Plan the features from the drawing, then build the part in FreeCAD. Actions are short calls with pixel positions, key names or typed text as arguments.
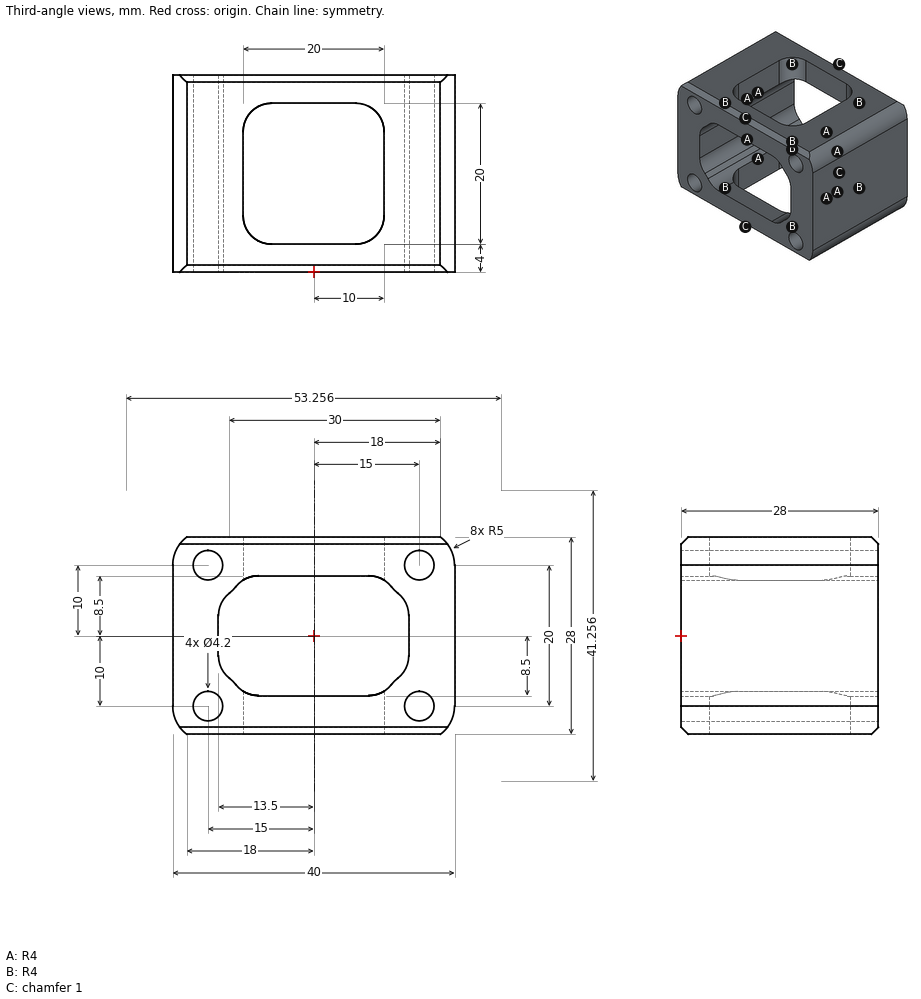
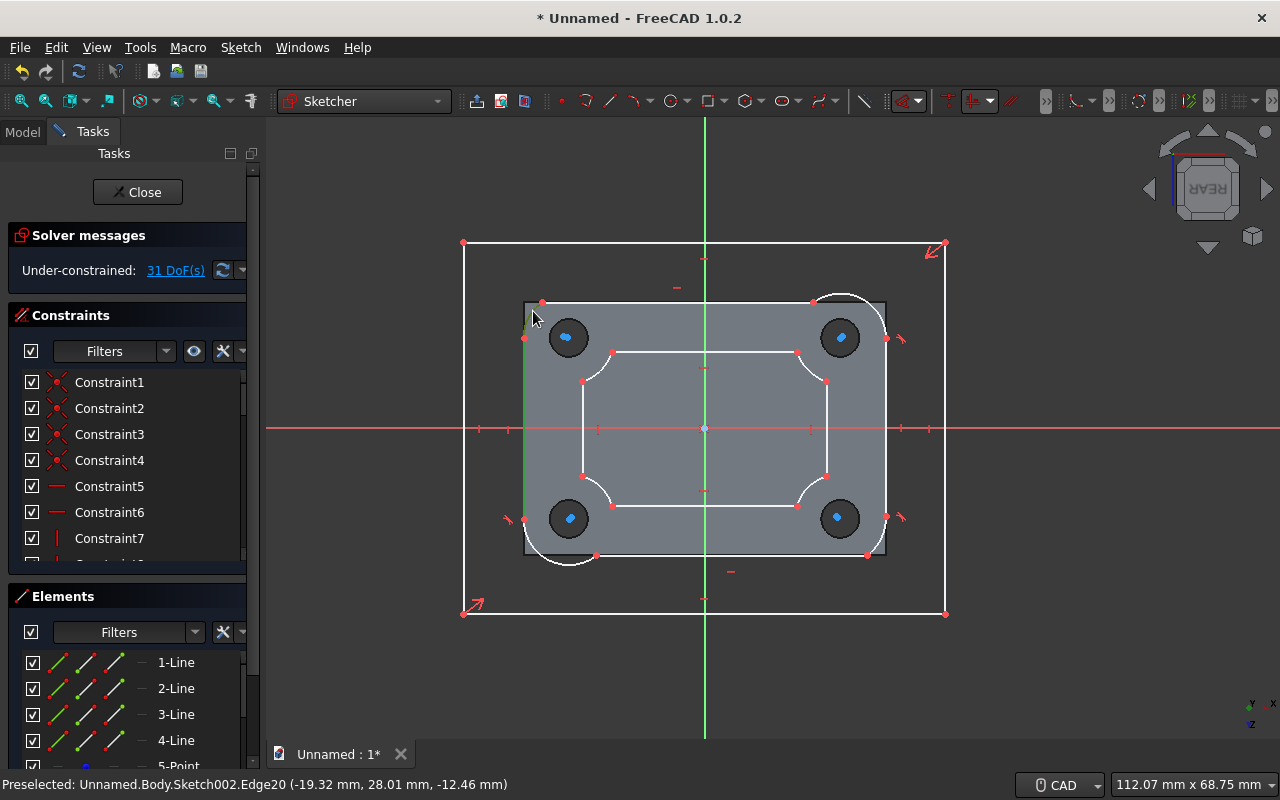
key(t)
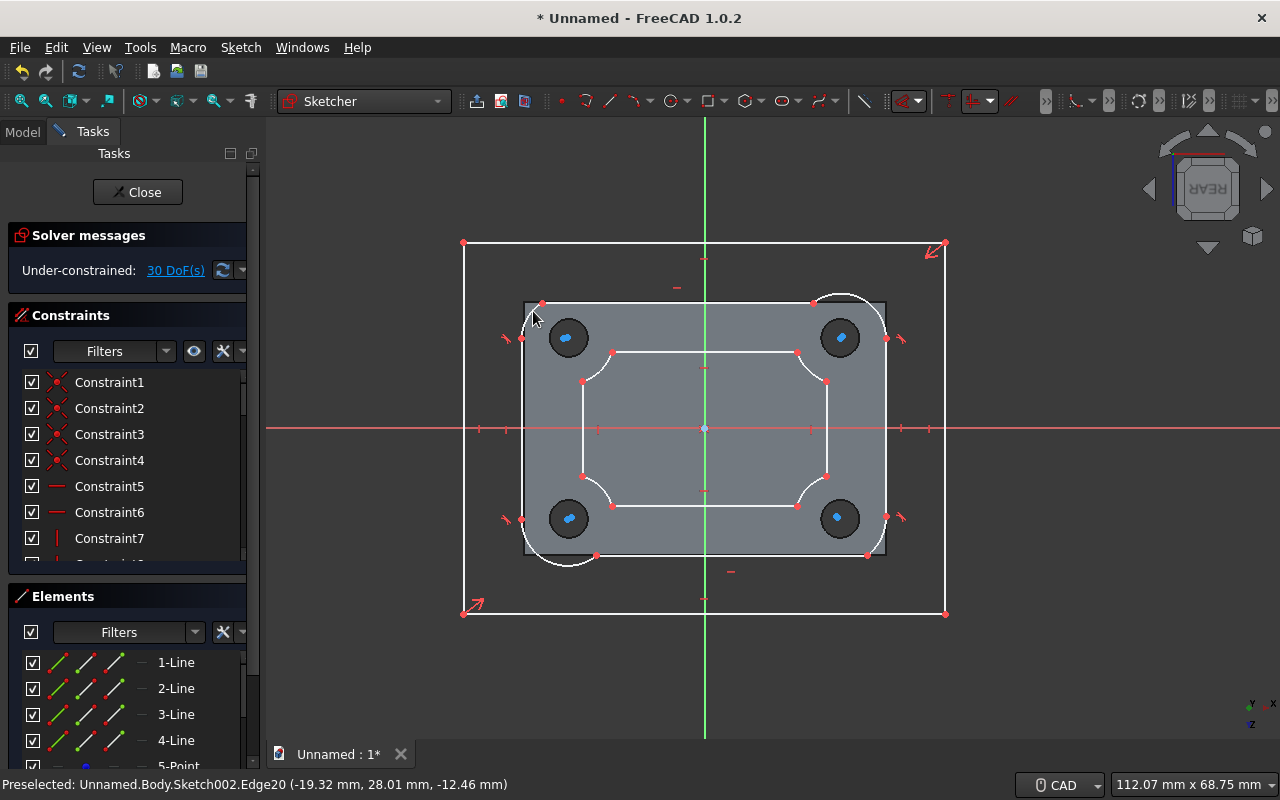
click(815, 482)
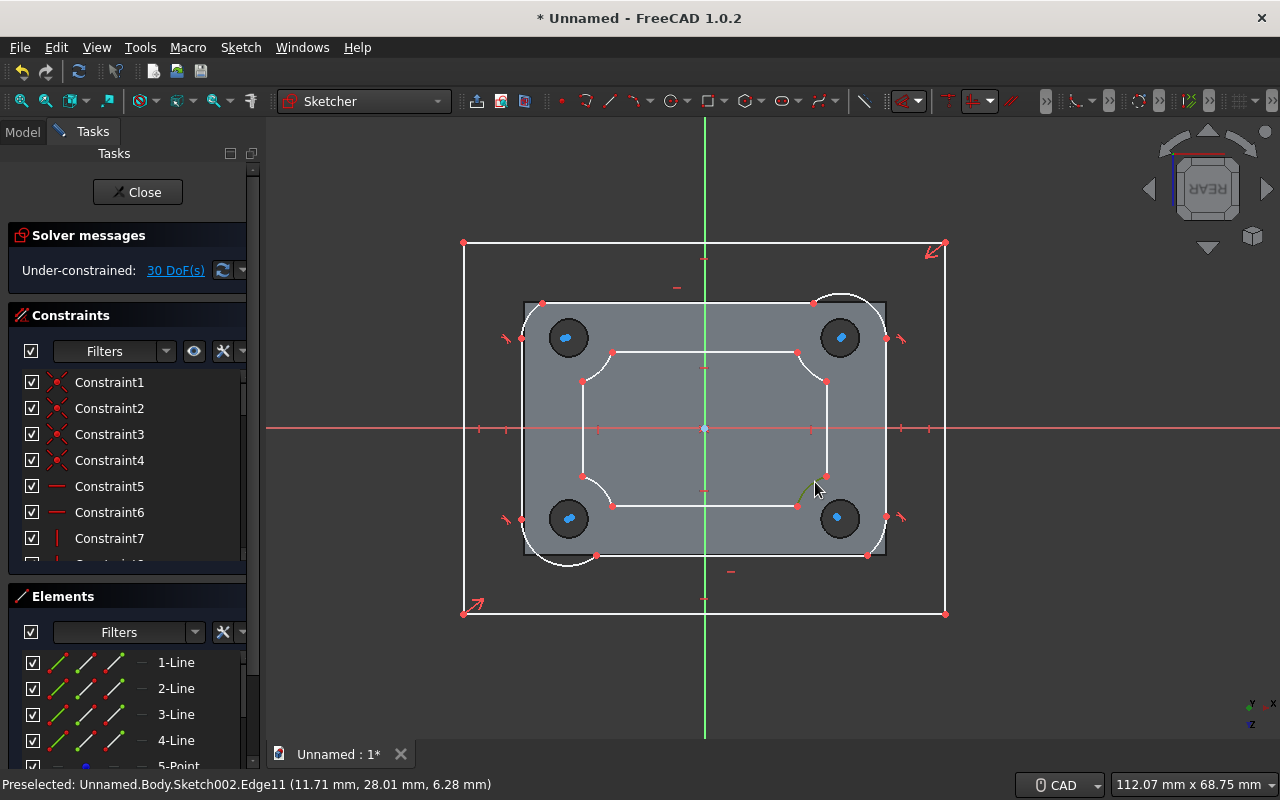
click(876, 546)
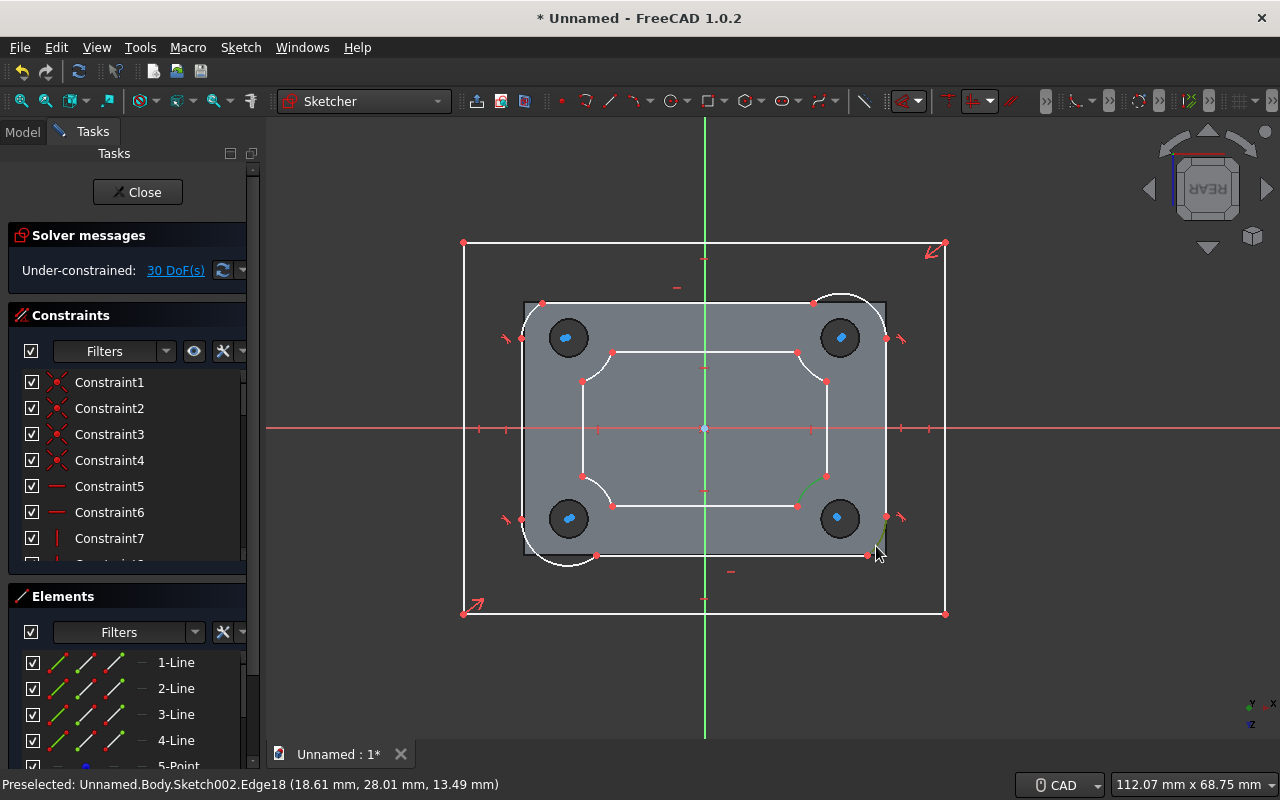
key(c)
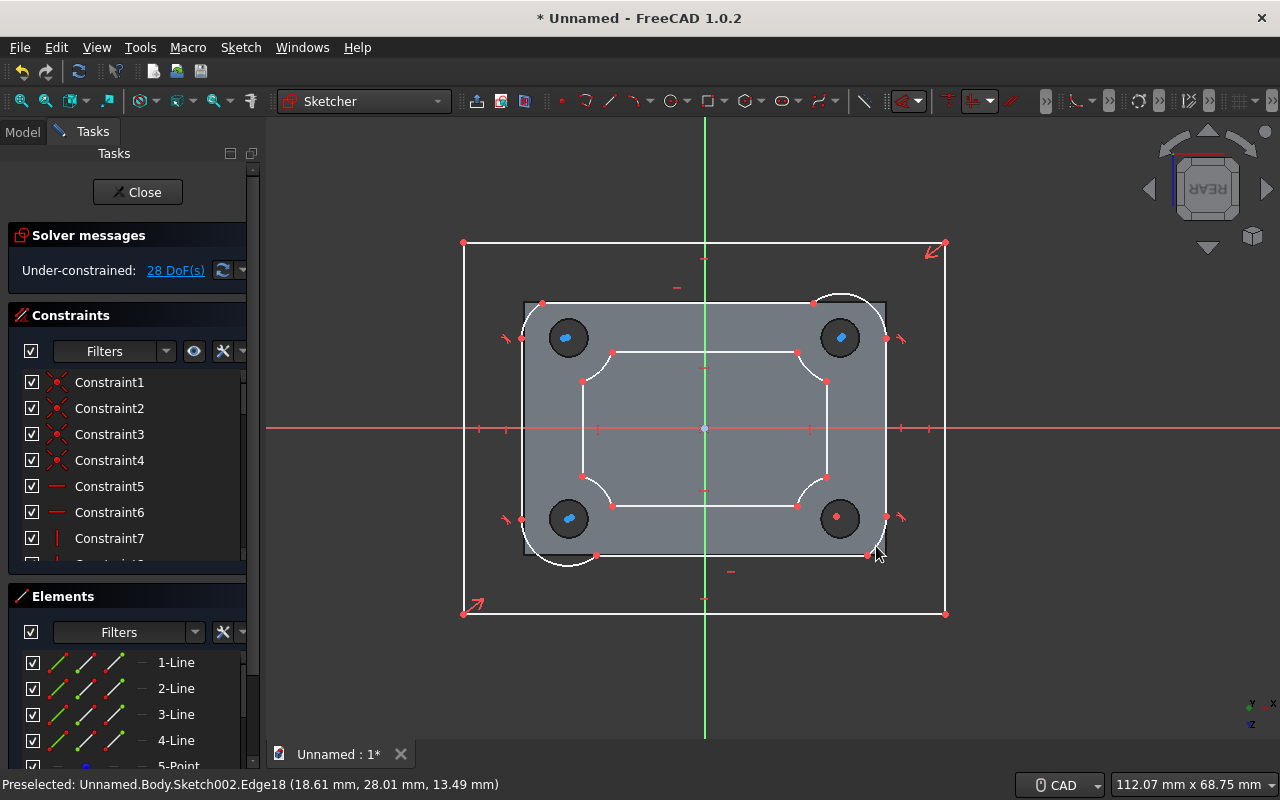
click(607, 494)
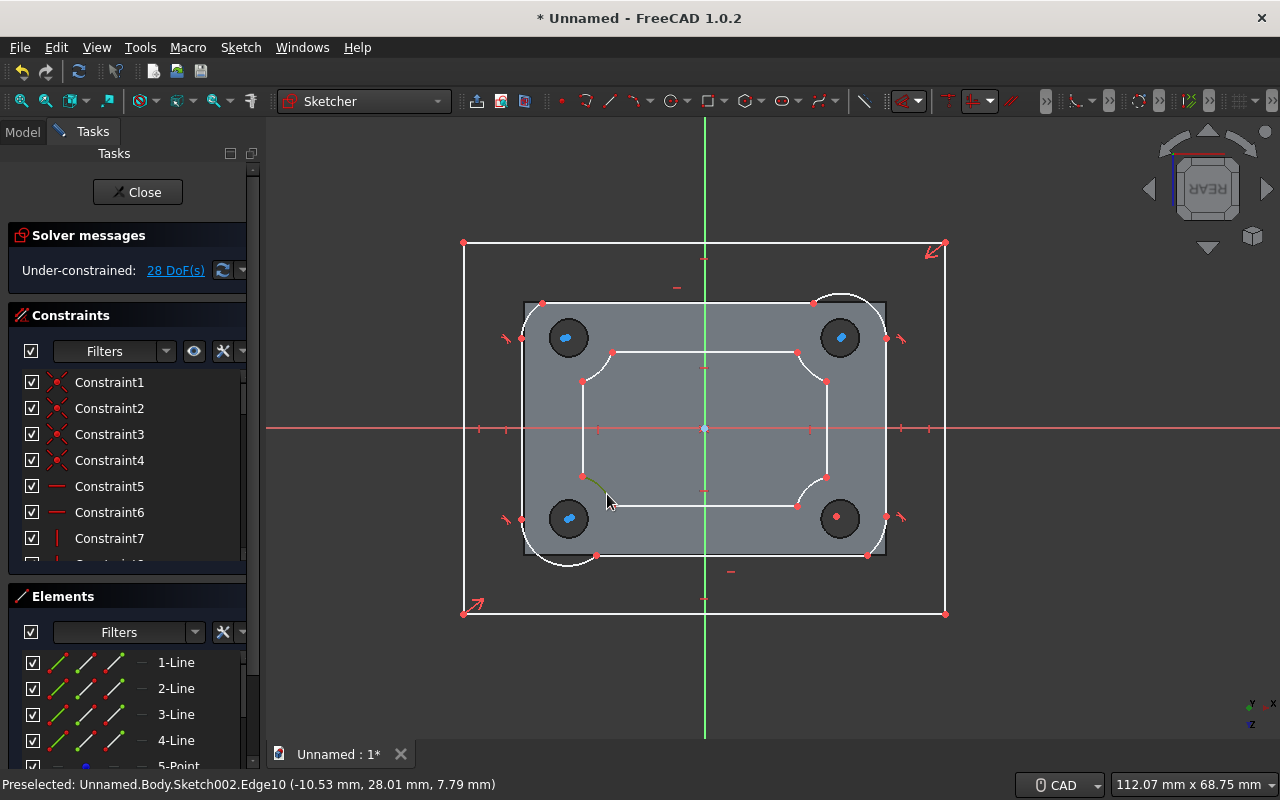
click(532, 549)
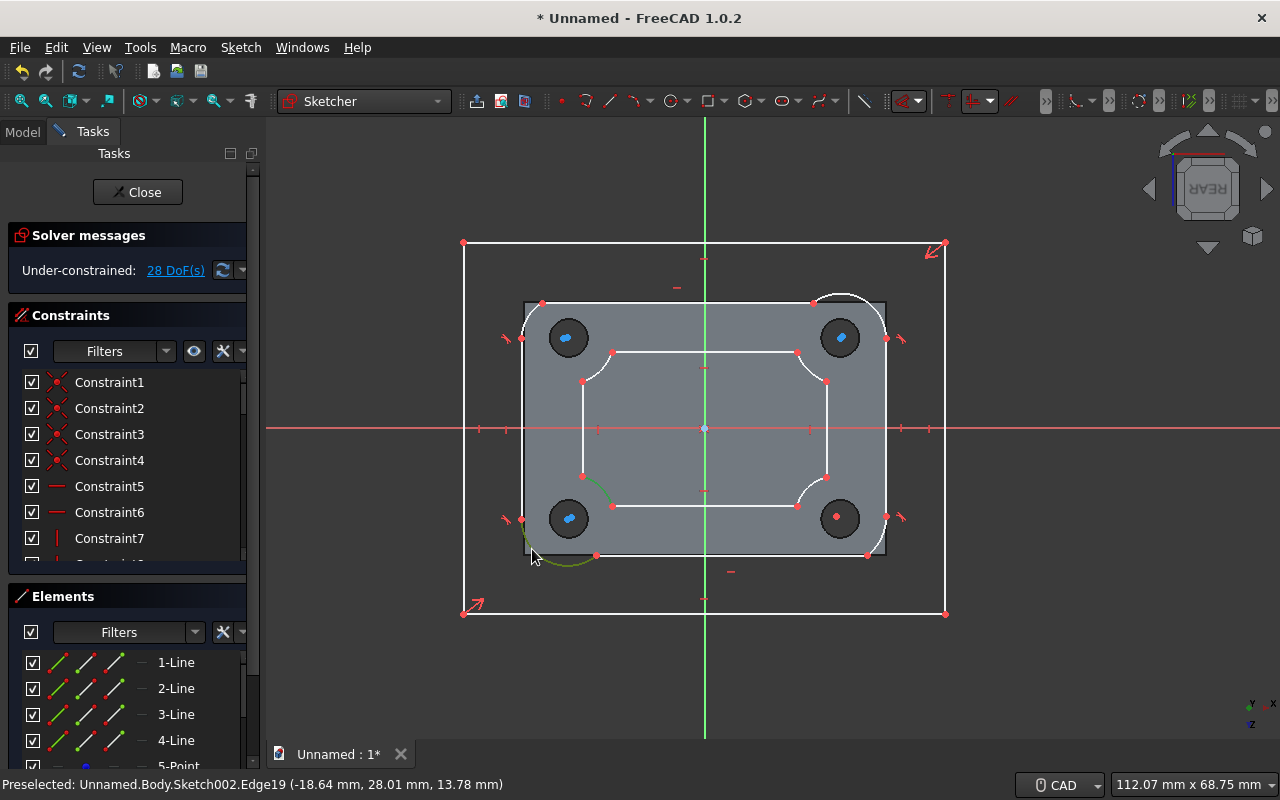
key(c)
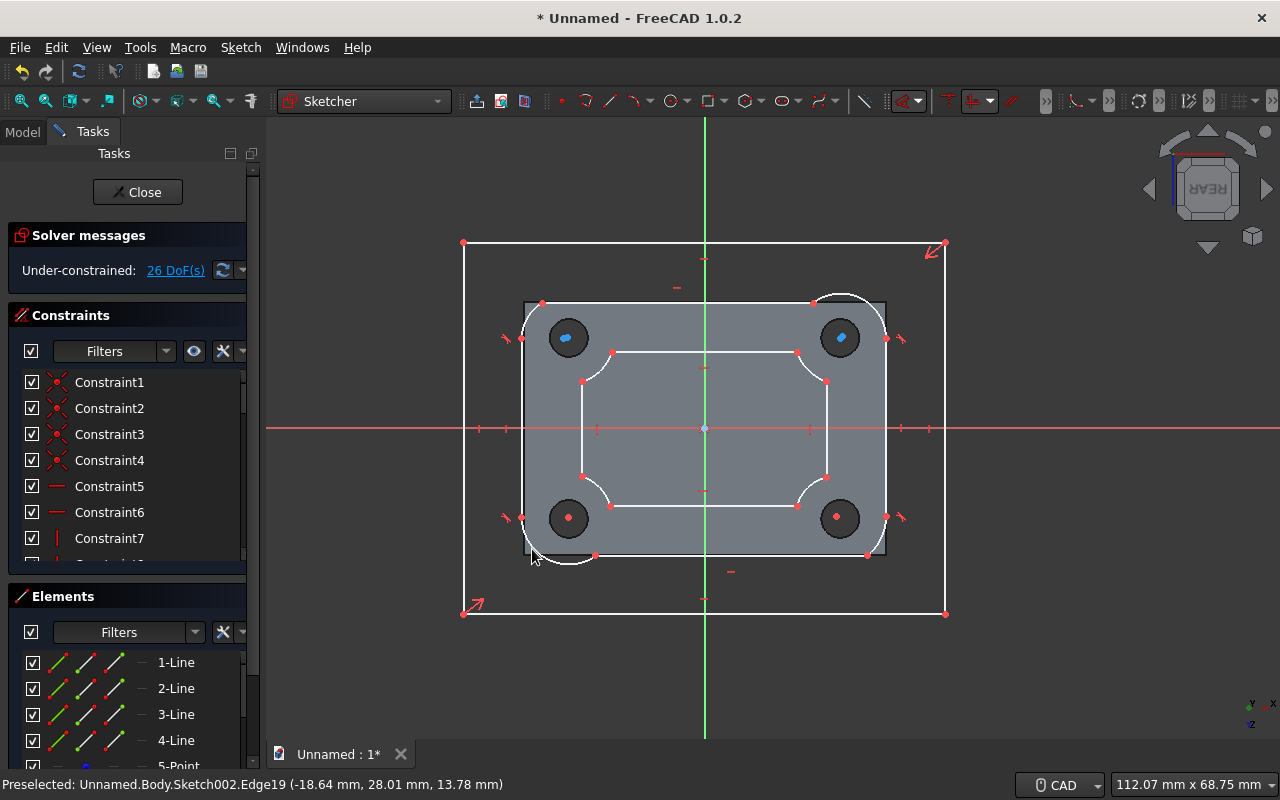
click(594, 376)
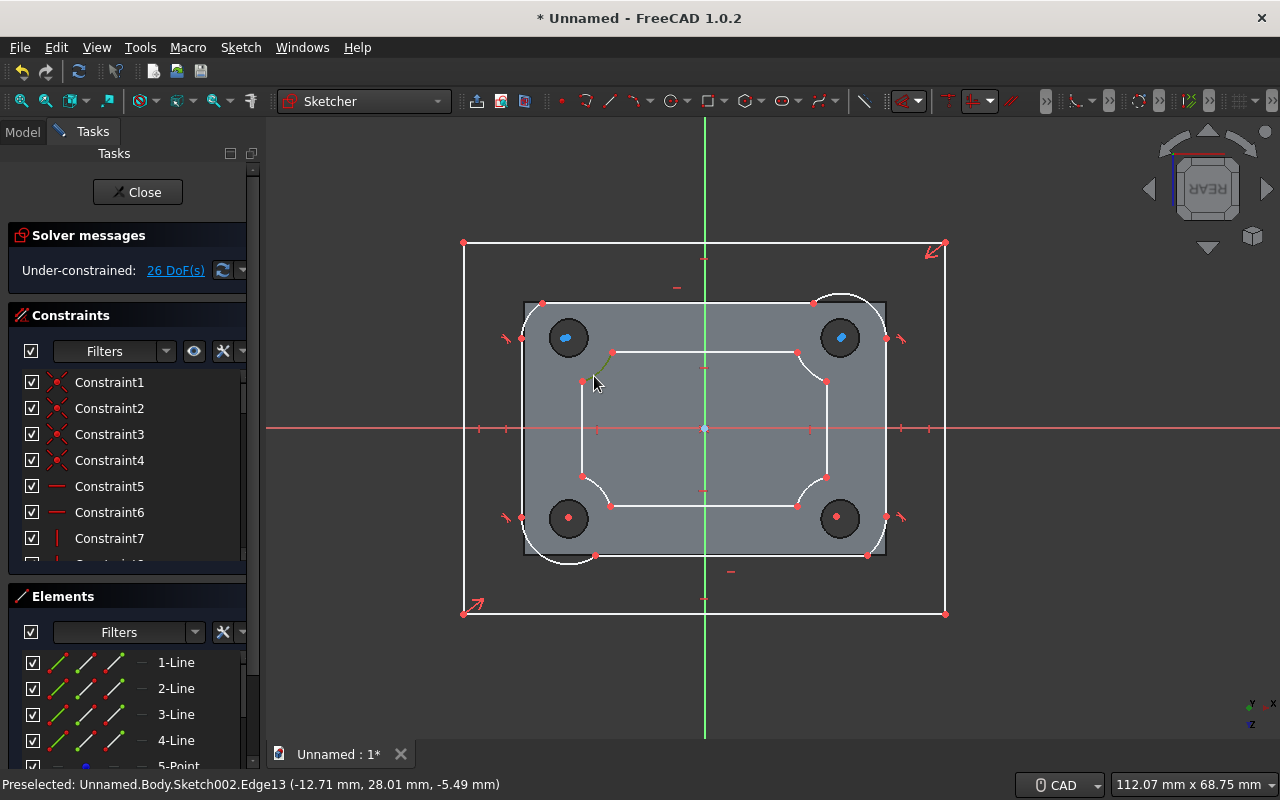
click(532, 311)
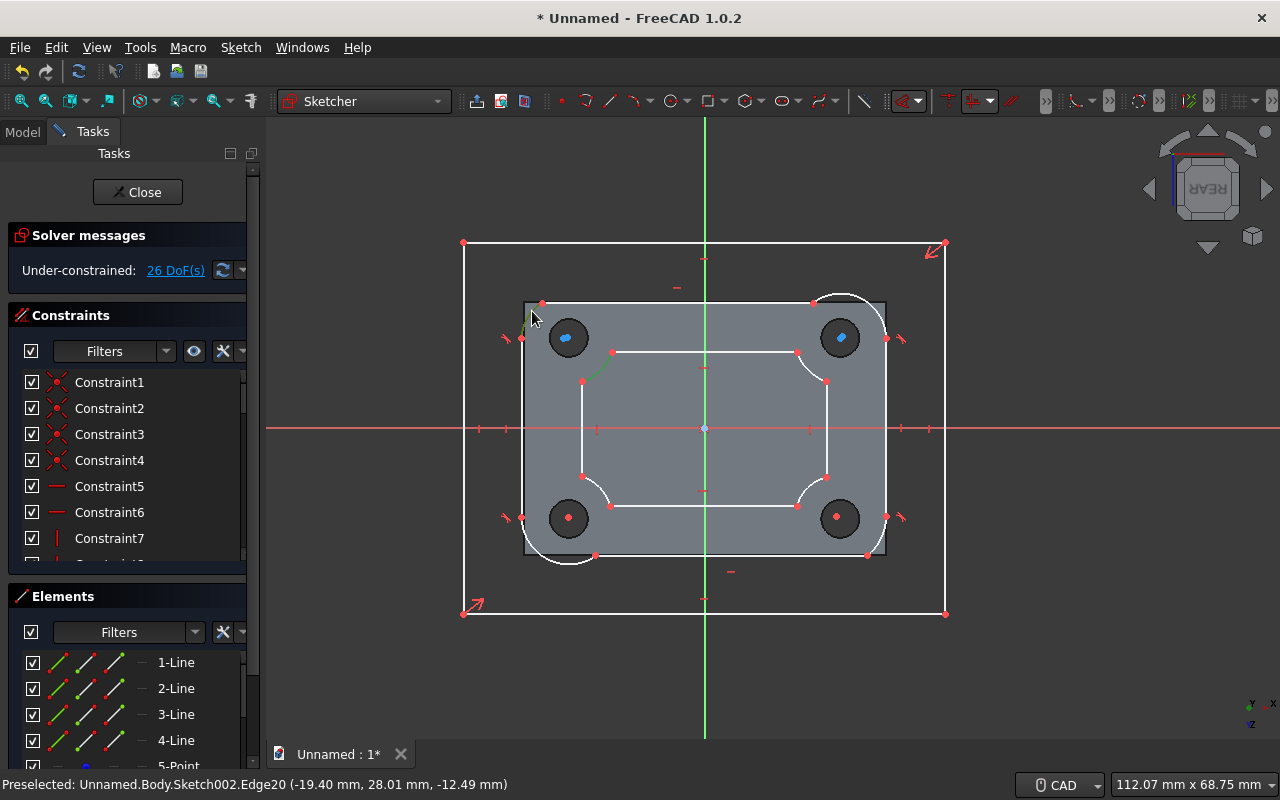
key(c)